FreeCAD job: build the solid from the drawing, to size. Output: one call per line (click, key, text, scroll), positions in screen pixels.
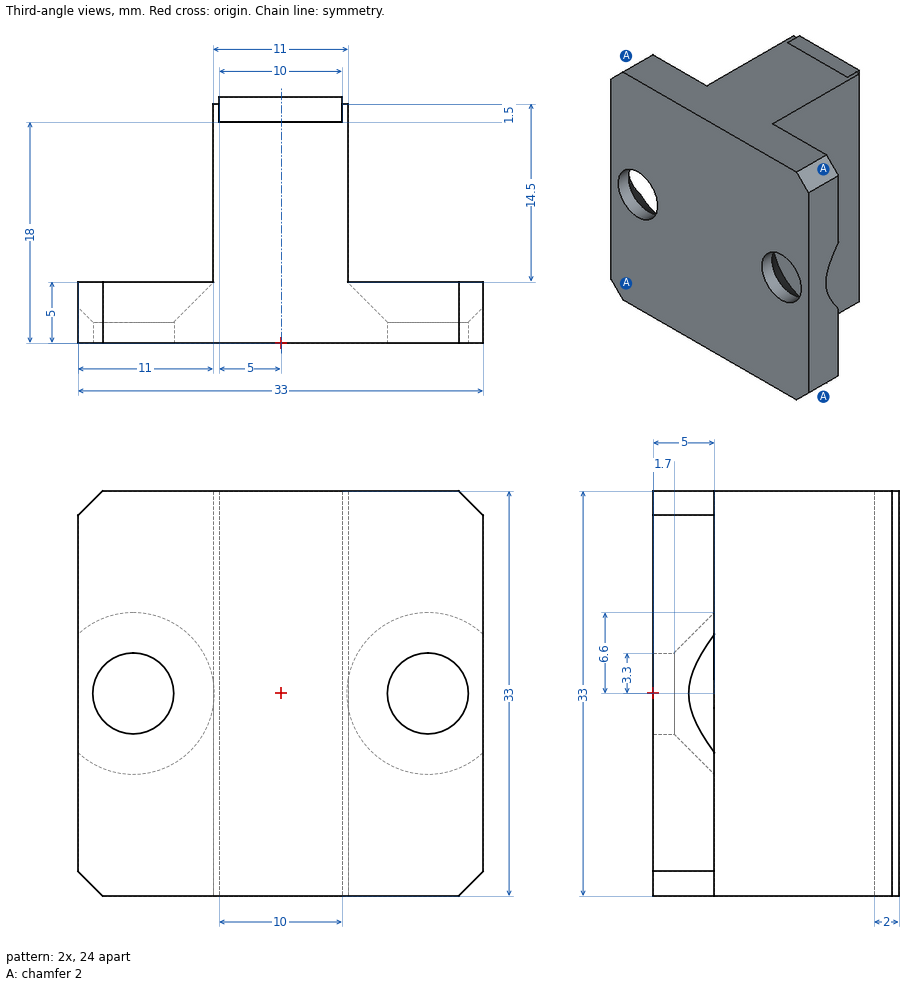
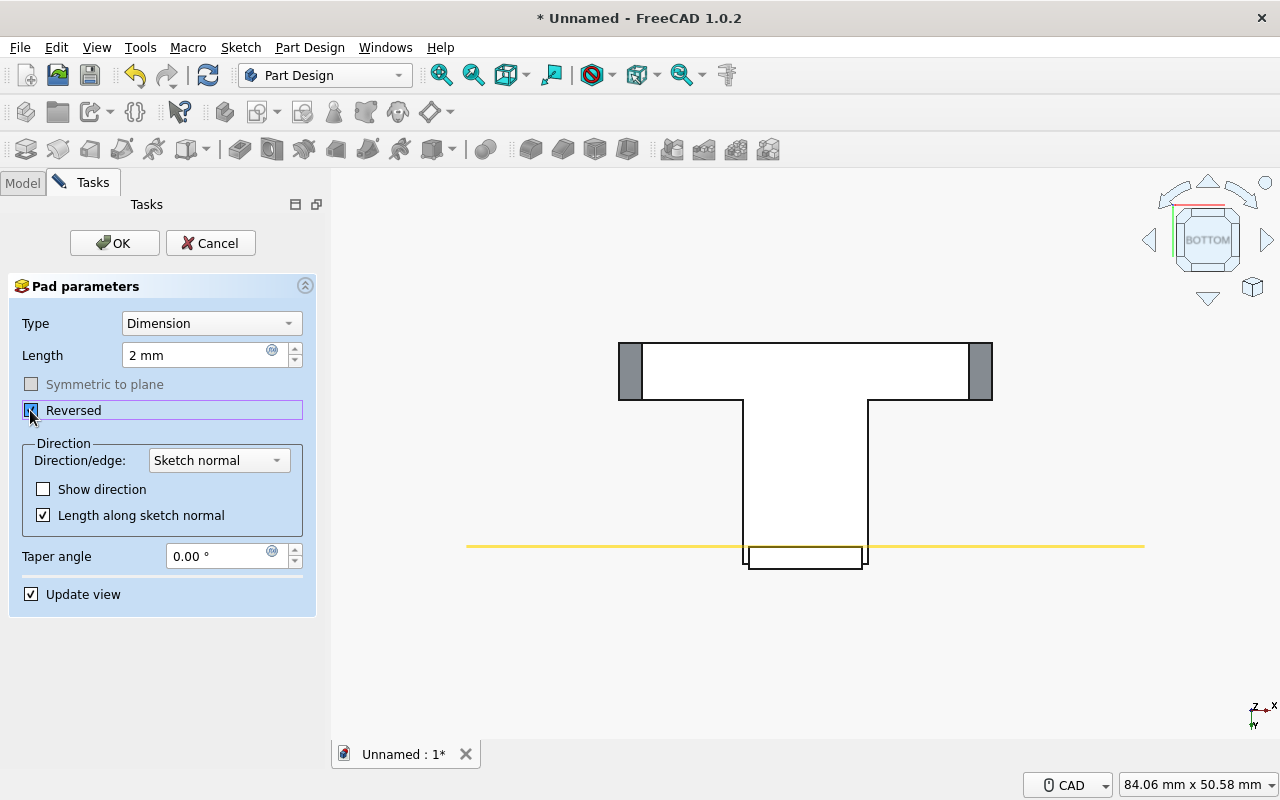
click(115, 243)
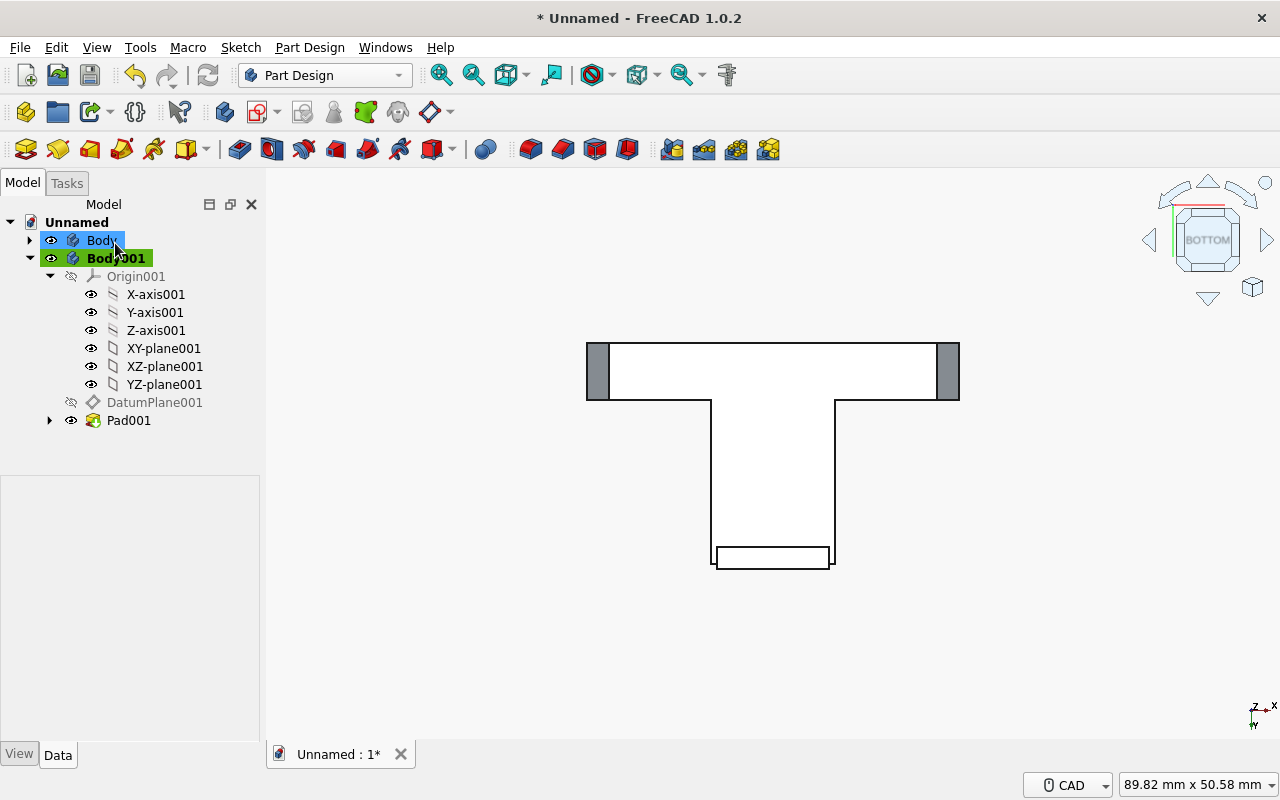
key(0)